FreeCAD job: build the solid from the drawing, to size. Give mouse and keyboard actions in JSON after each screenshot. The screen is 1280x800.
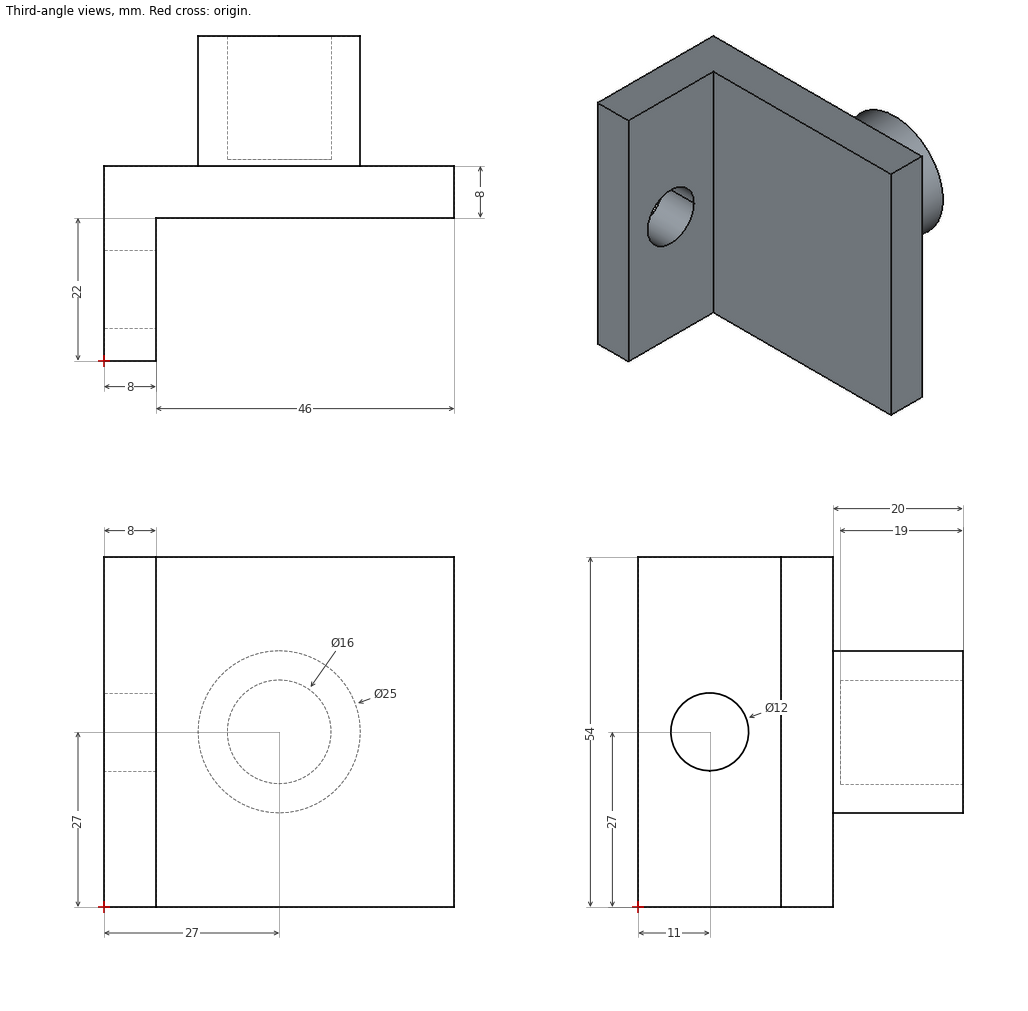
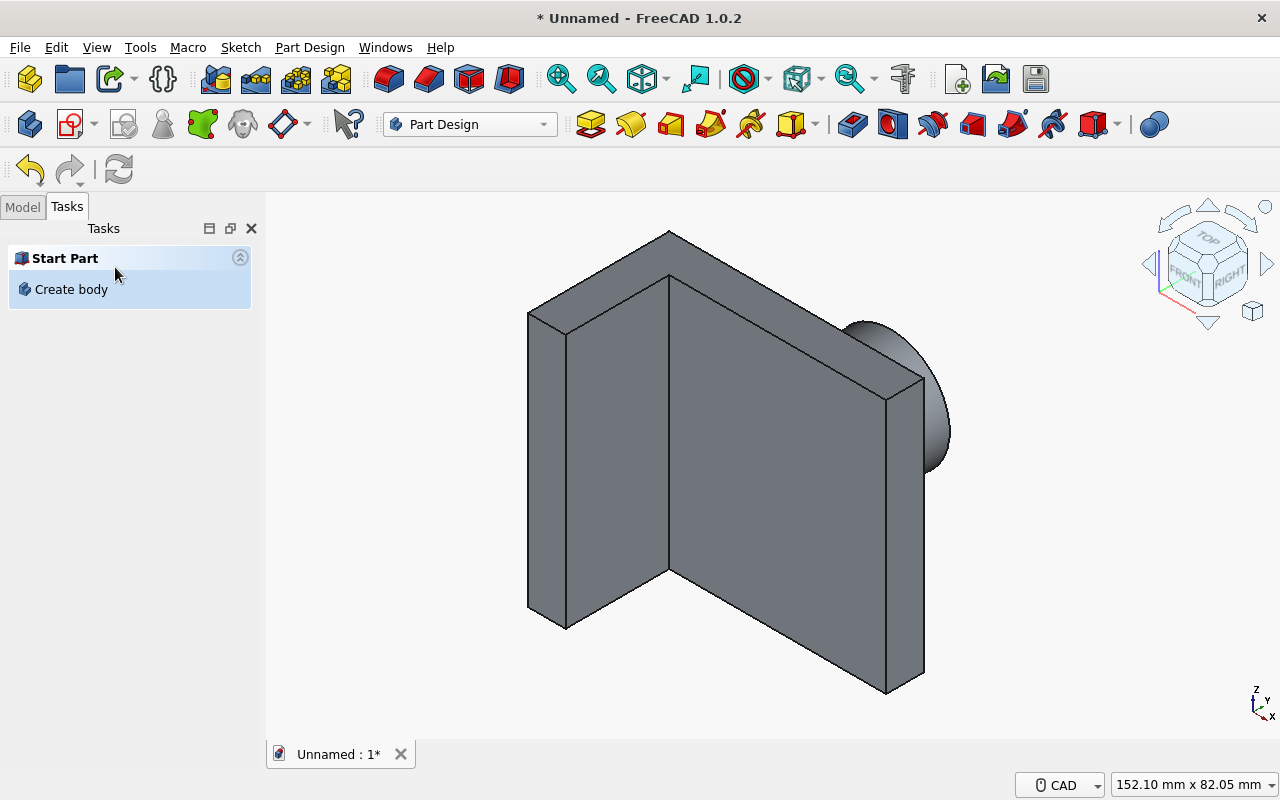
{"action": "left_click", "coordinate": [562, 80]}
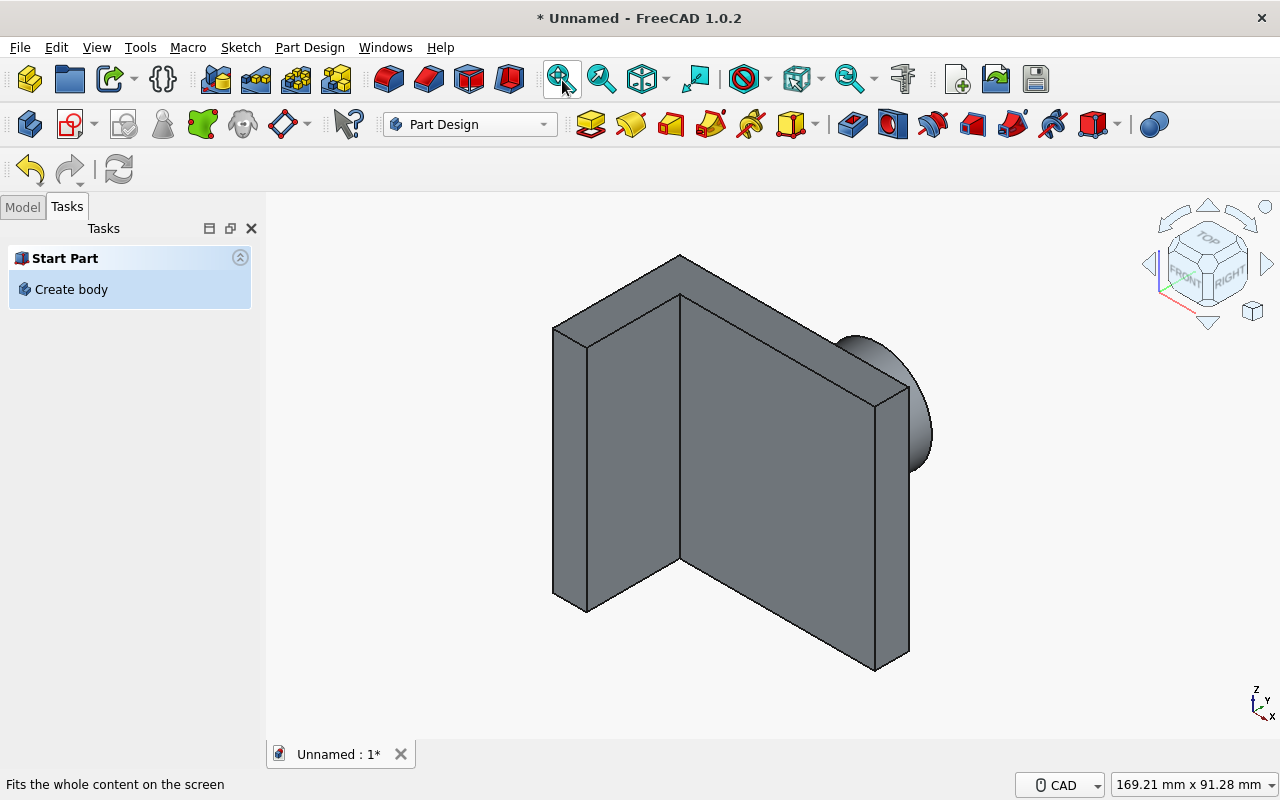
{"action": "left_click", "coordinate": [633, 377]}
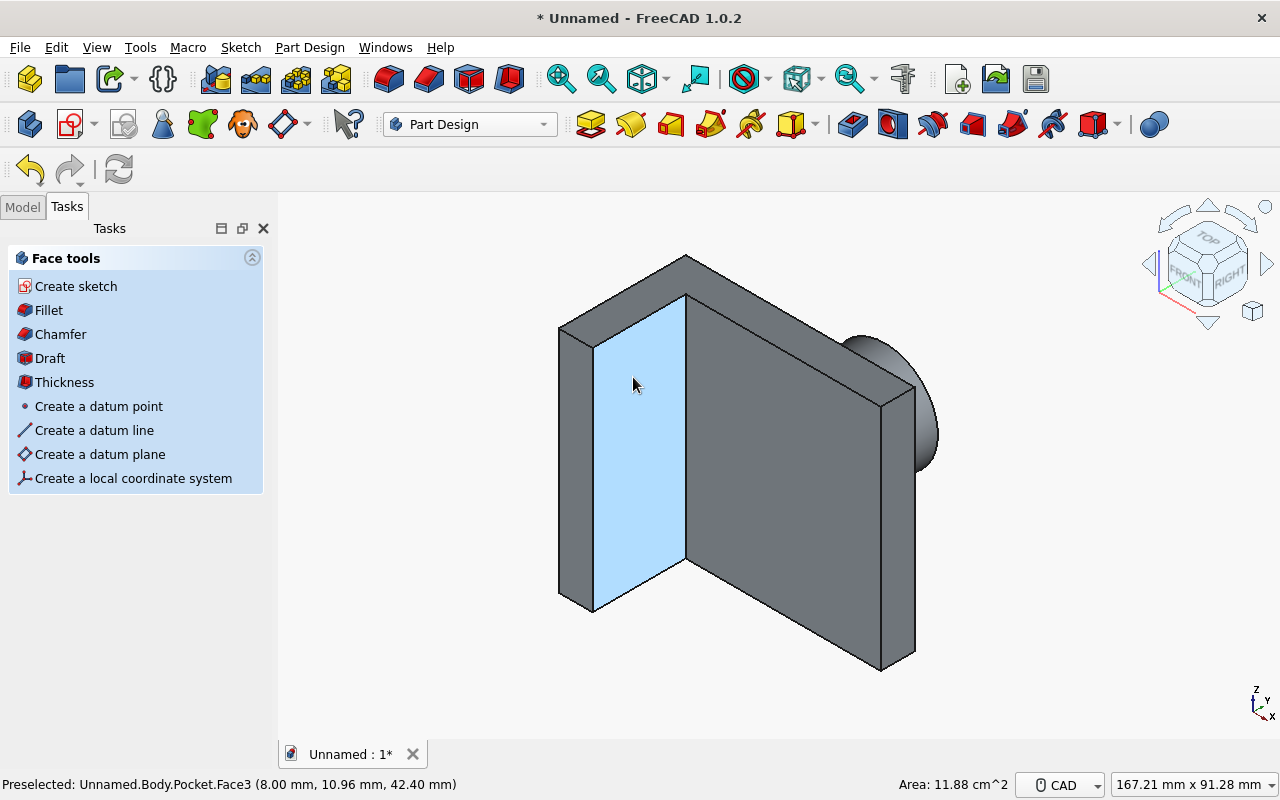
{"action": "left_click", "coordinate": [70, 124]}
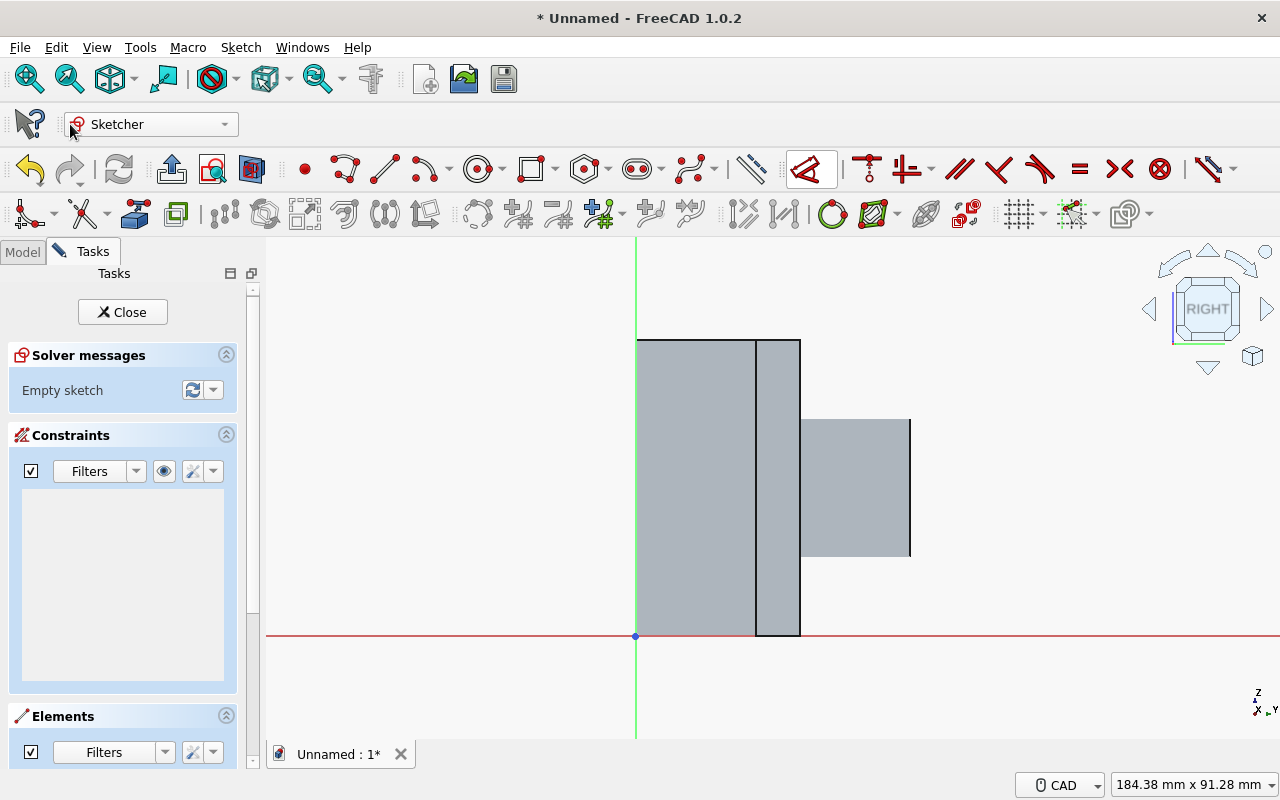
{"action": "key", "text": "q s"}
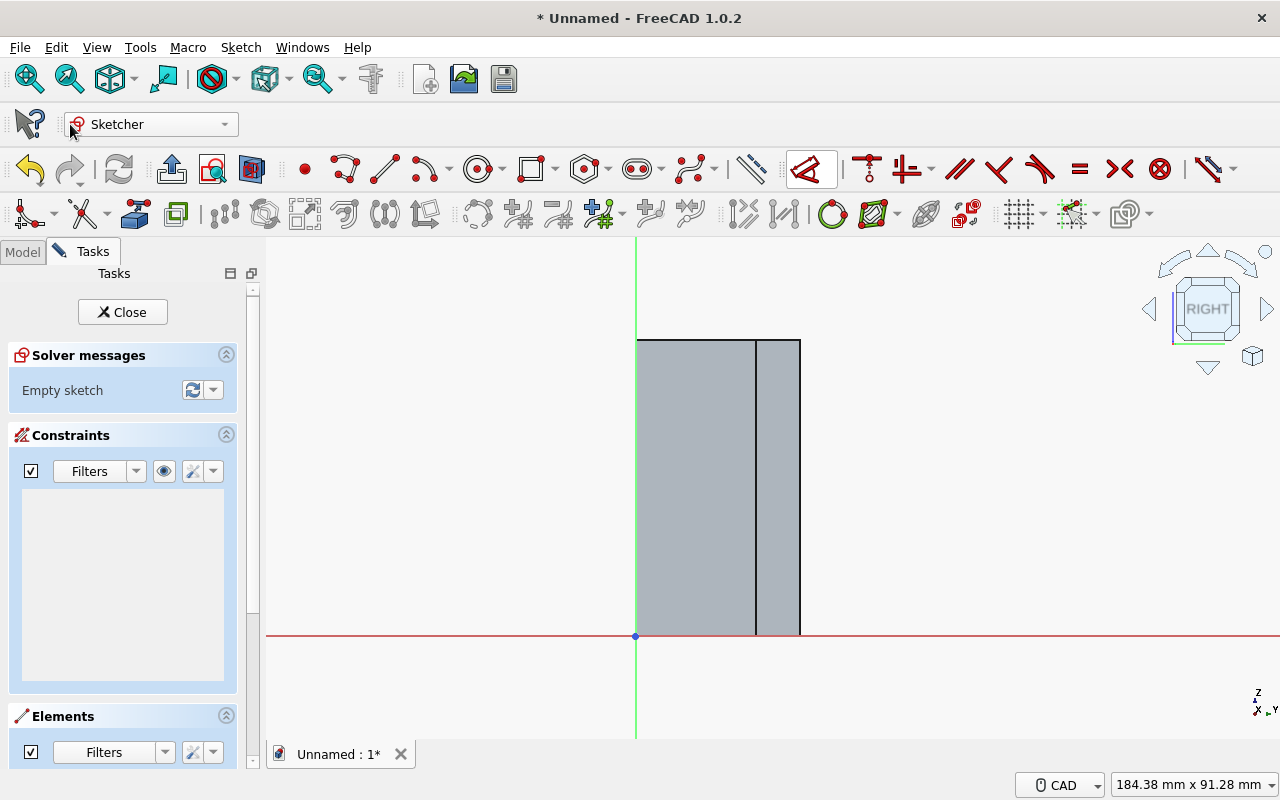
{"action": "scroll", "coordinate": [694, 488], "scroll_direction": "up", "scroll_amount": 8}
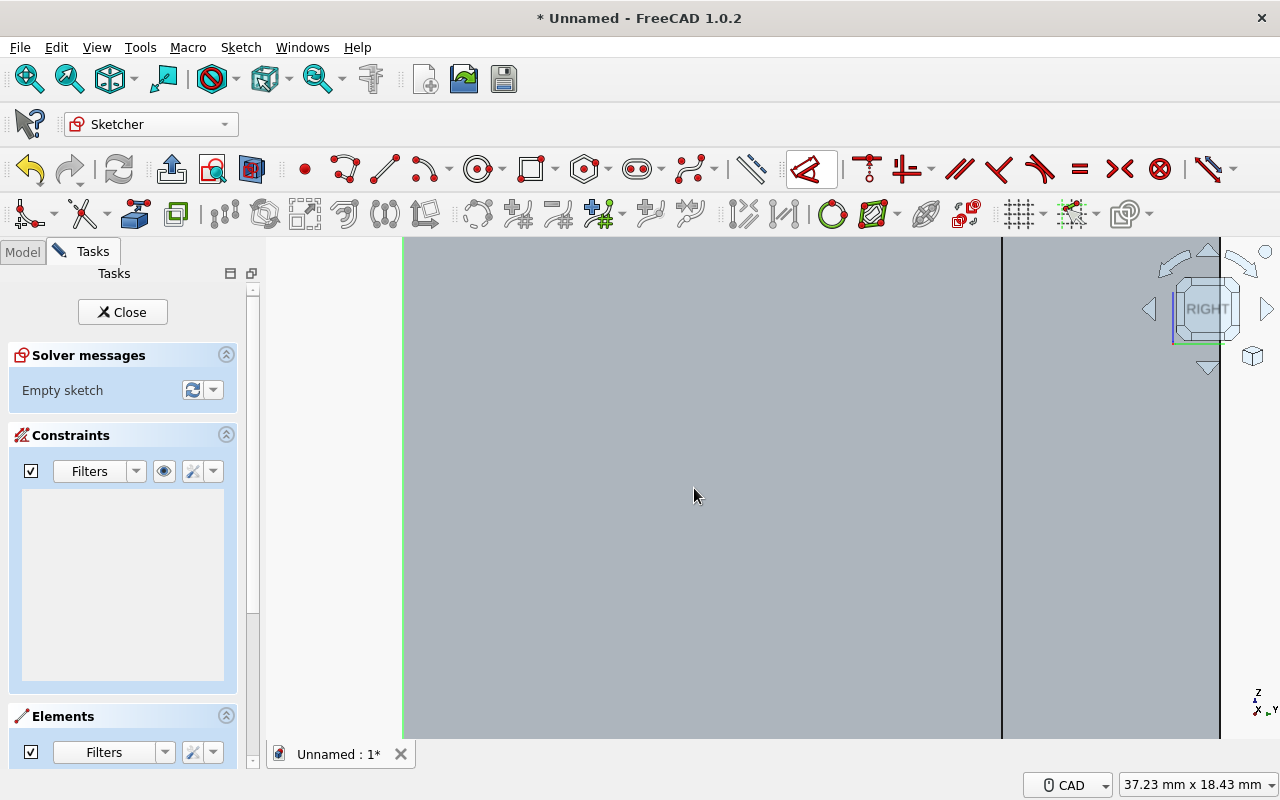
{"action": "key", "text": "g c"}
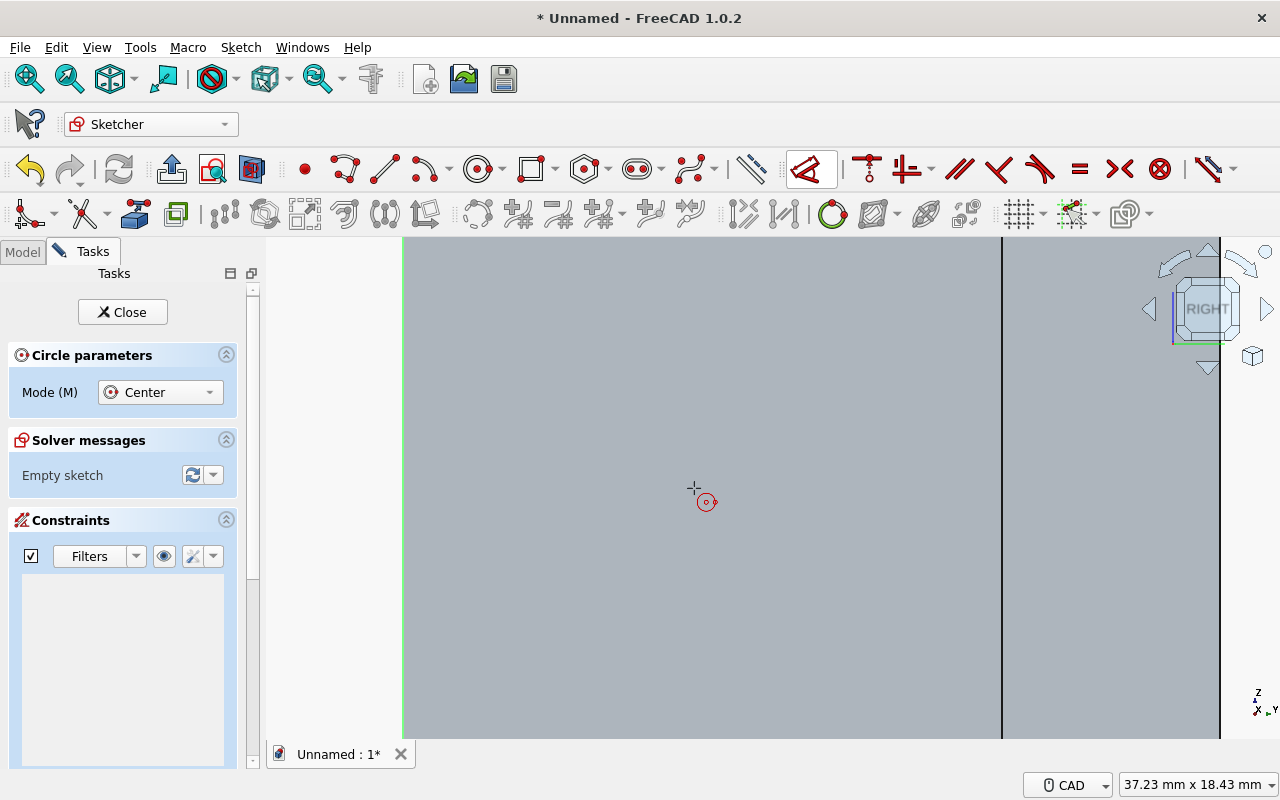
{"action": "left_click", "coordinate": [702, 486]}
{"action": "mouse_move", "coordinate": [818, 370]}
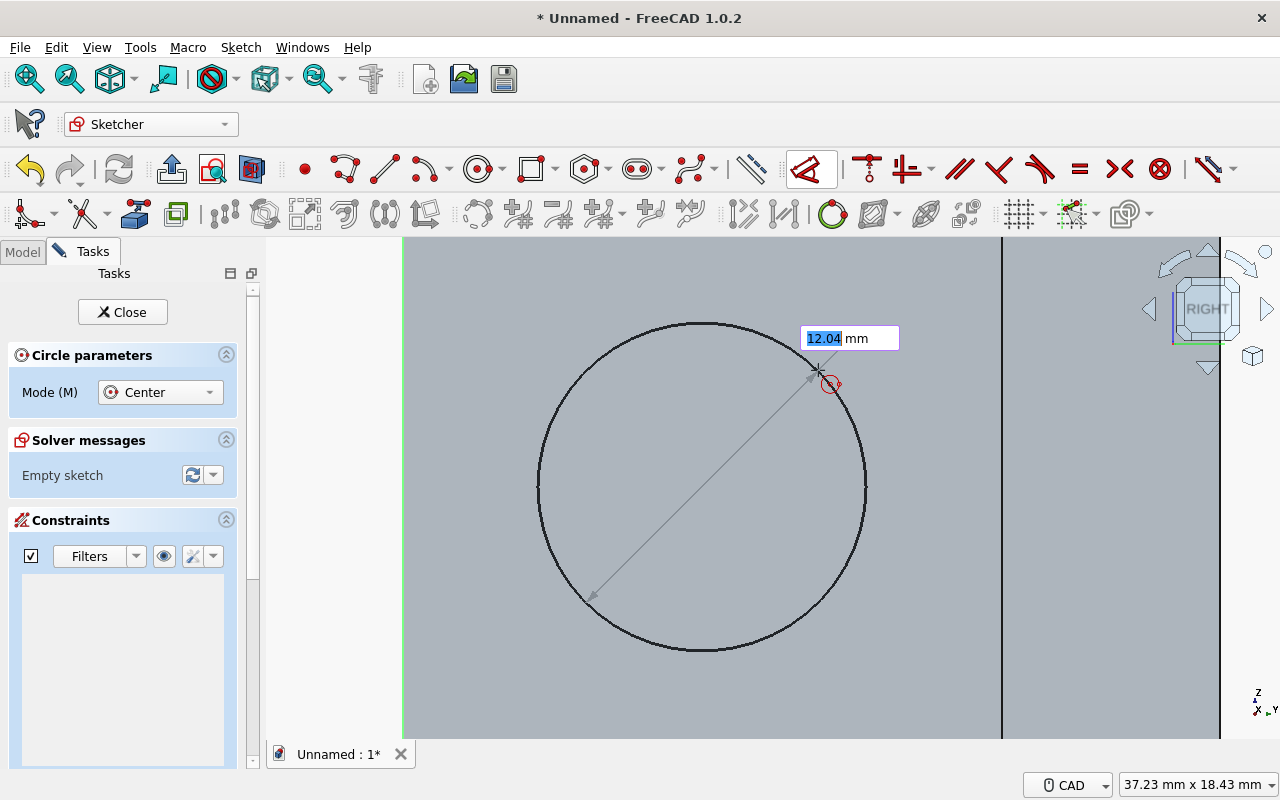
{"action": "type", "text": "12"}
{"action": "key", "text": "Return"}
{"action": "key", "text": "Escape"}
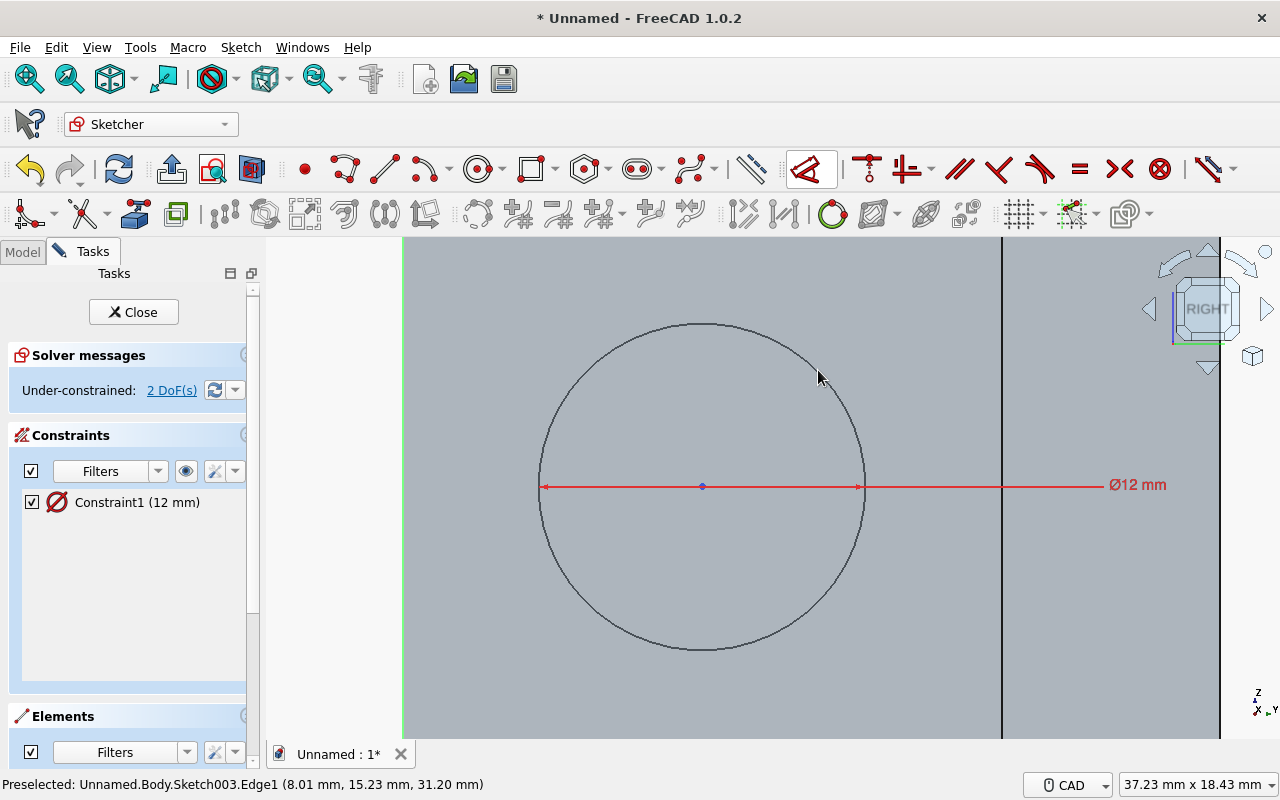
{"action": "left_click", "coordinate": [702, 487]}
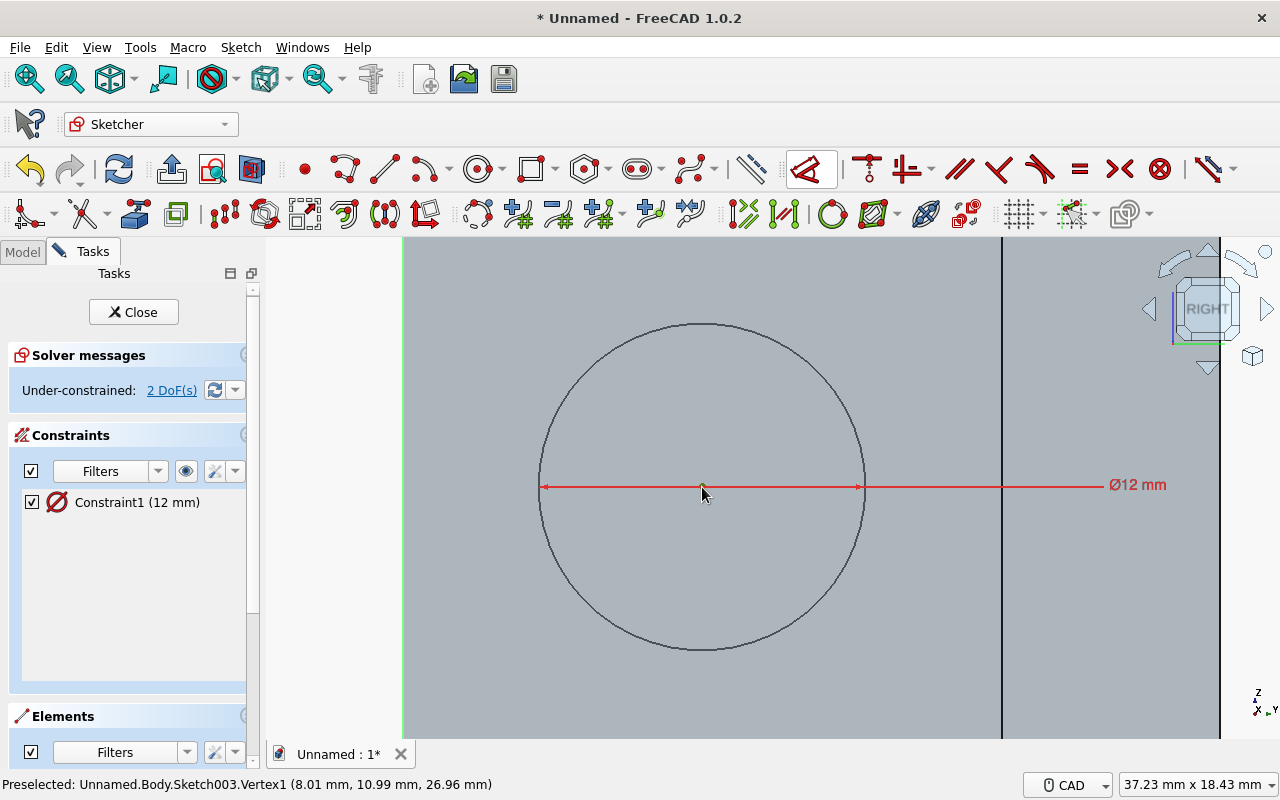
{"action": "key", "text": "l"}